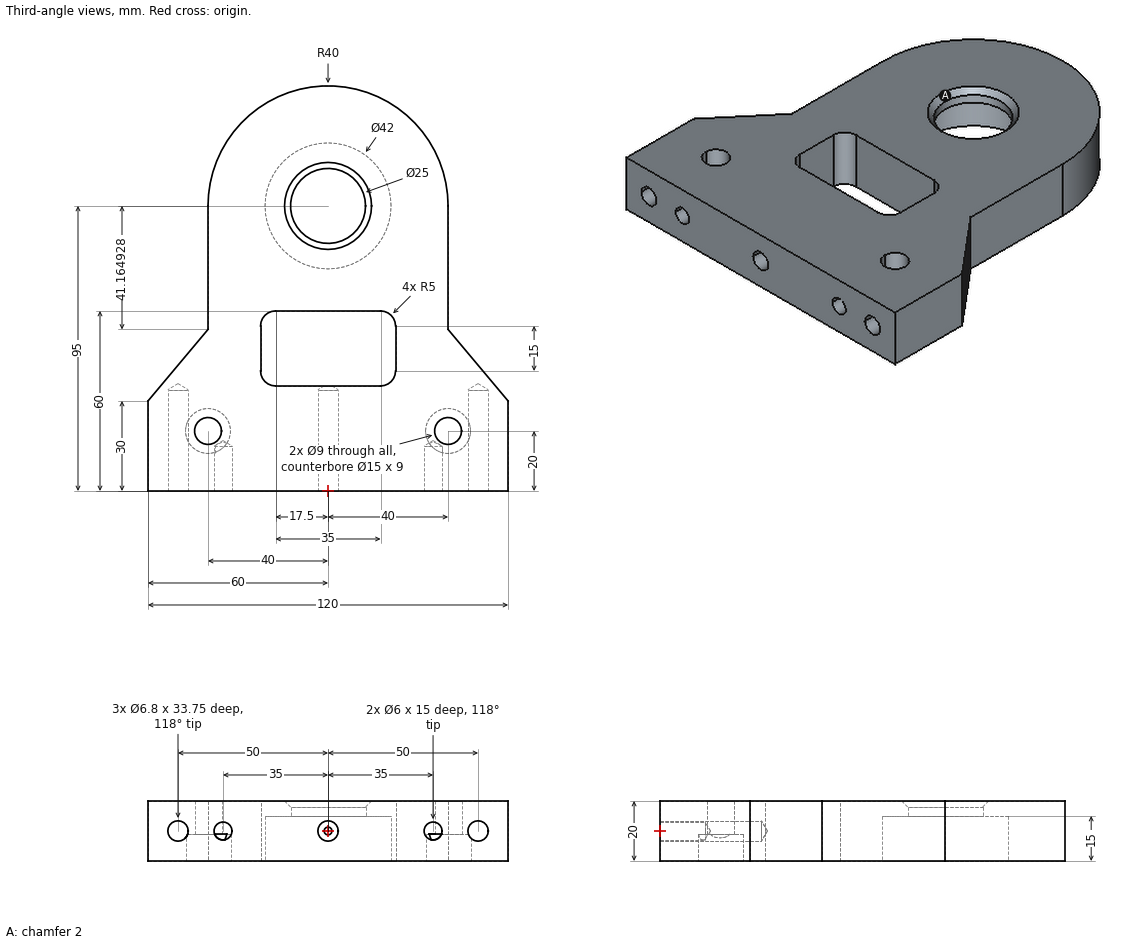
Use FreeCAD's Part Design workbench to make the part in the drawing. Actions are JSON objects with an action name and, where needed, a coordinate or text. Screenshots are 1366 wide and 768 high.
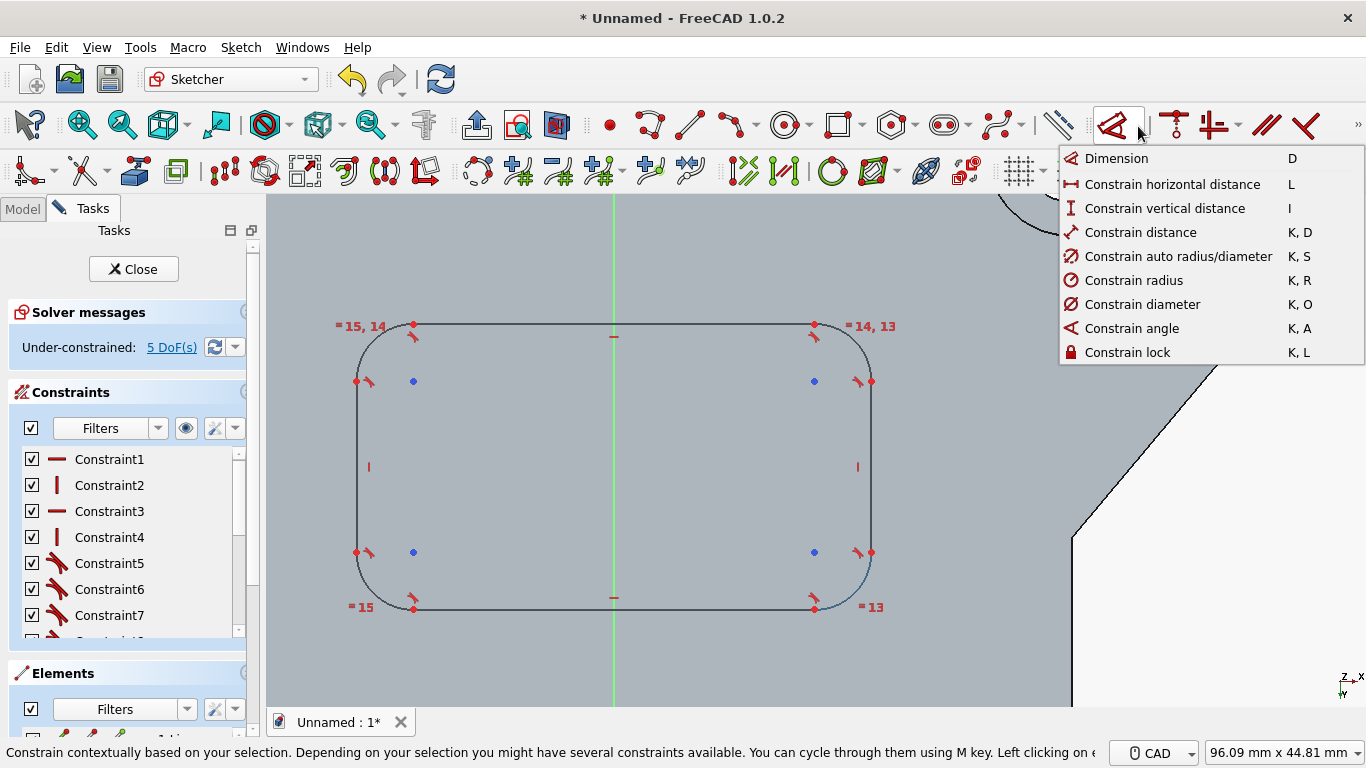
{"action": "left_click", "coordinate": [1212, 280]}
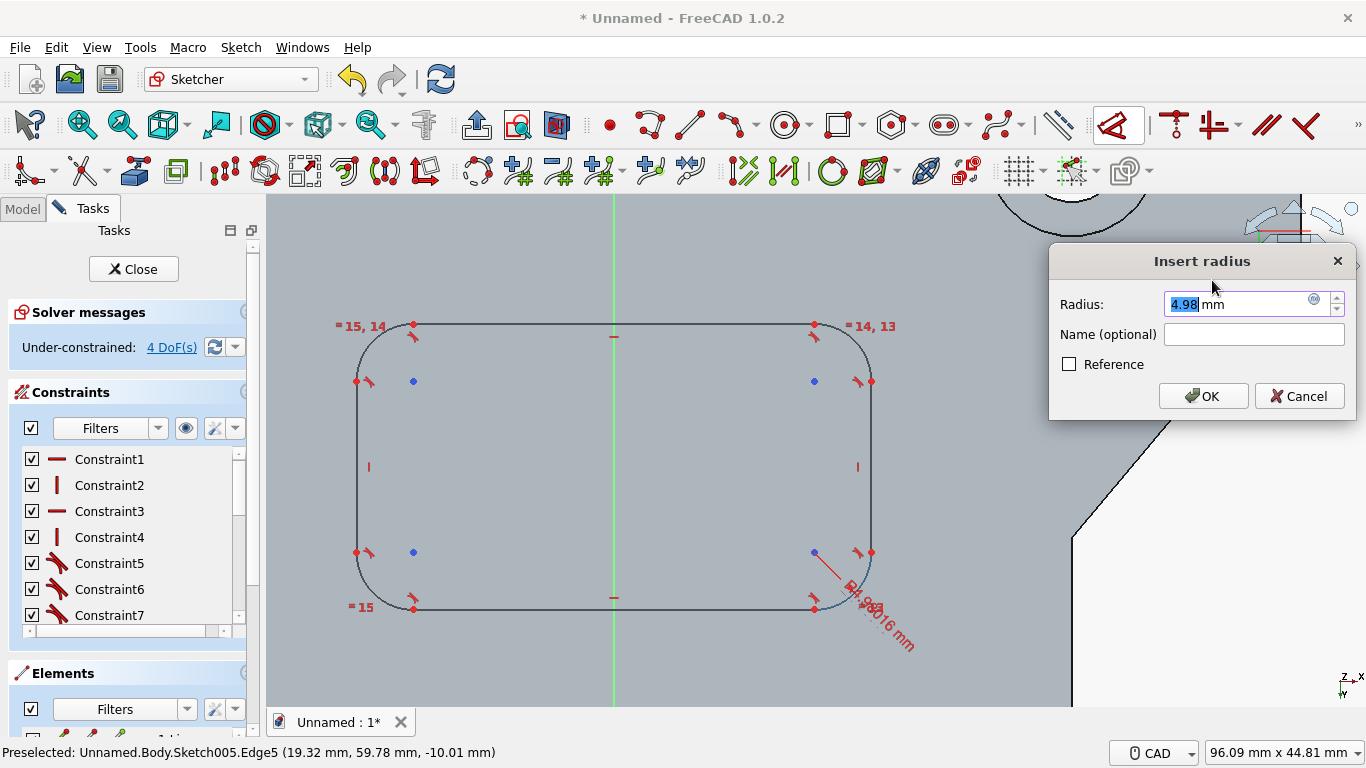
{"action": "type", "text": "5"}
{"action": "key", "text": "Return"}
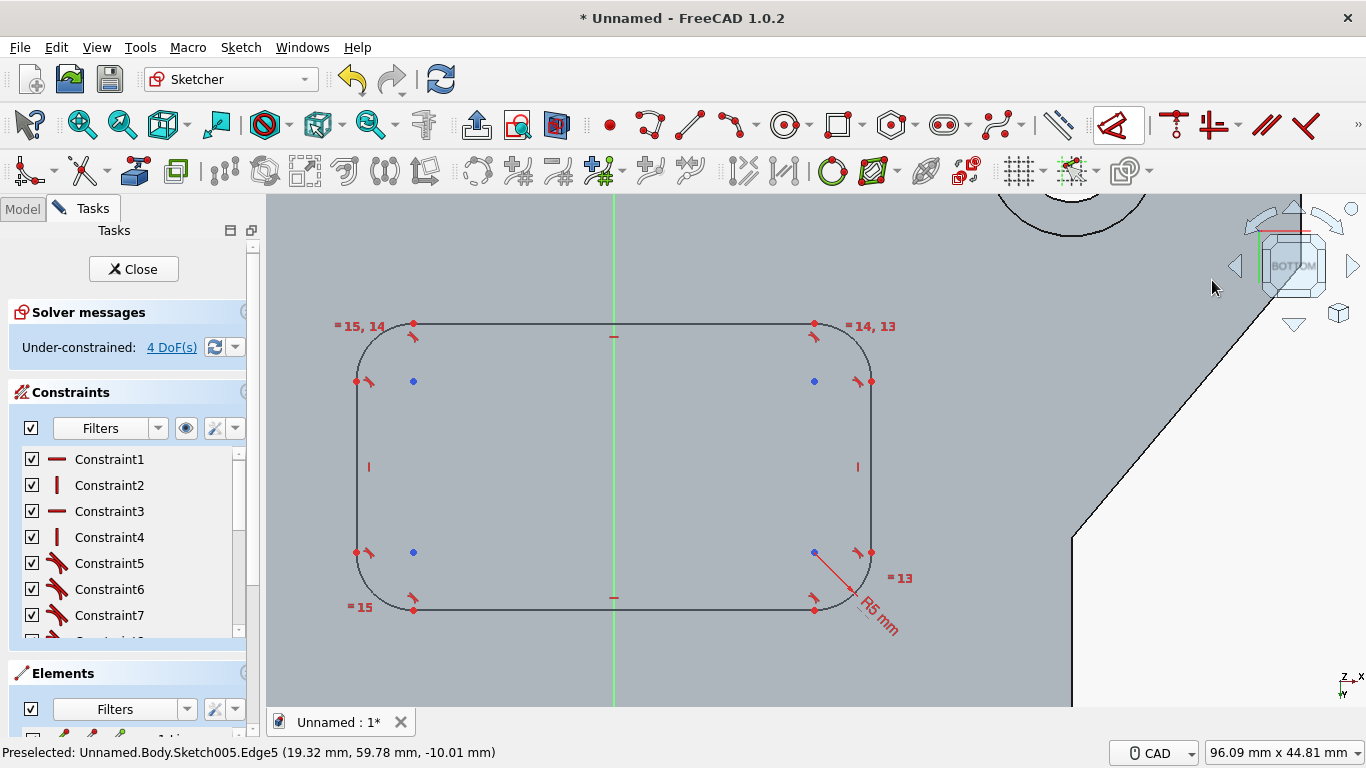
{"action": "left_click", "coordinate": [534, 610]}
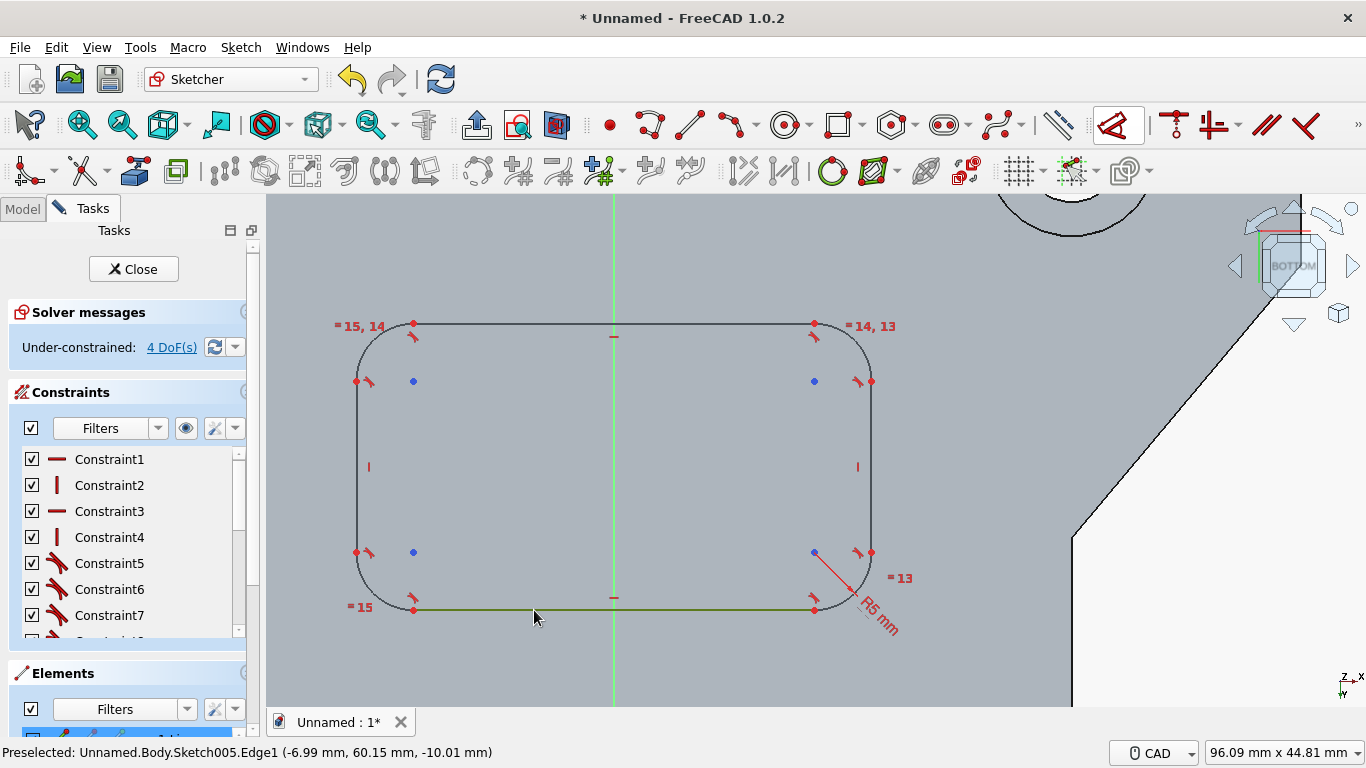
{"action": "key", "text": "l"}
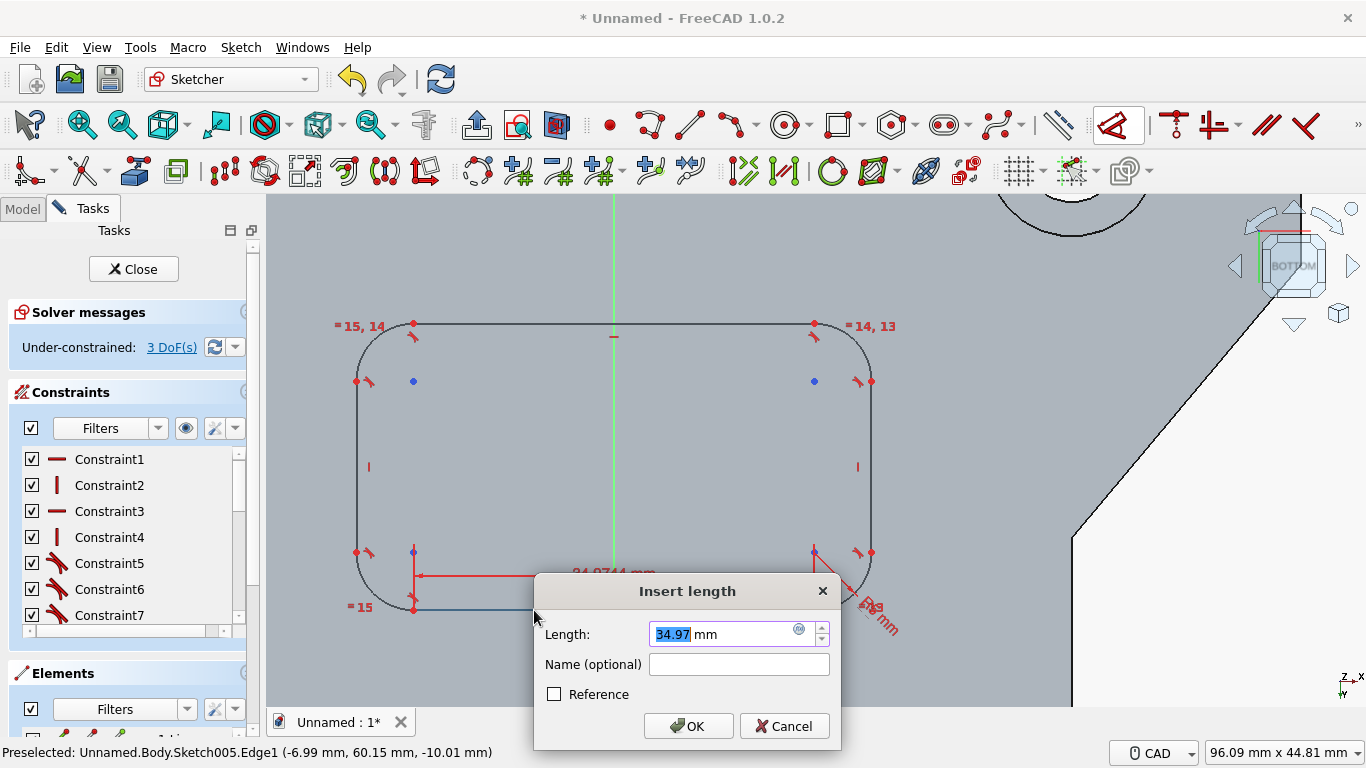
{"action": "type", "text": "35"}
{"action": "key", "text": "Return"}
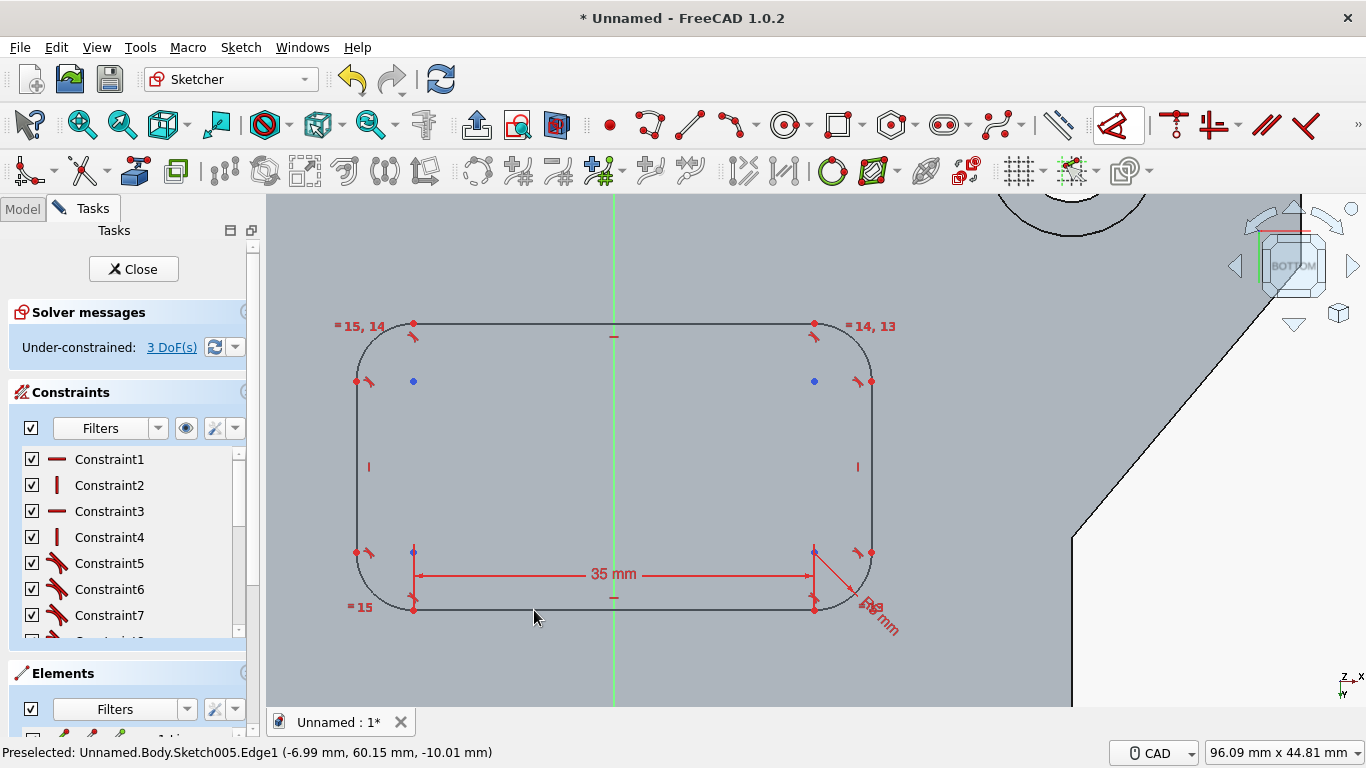
{"action": "left_click", "coordinate": [872, 501]}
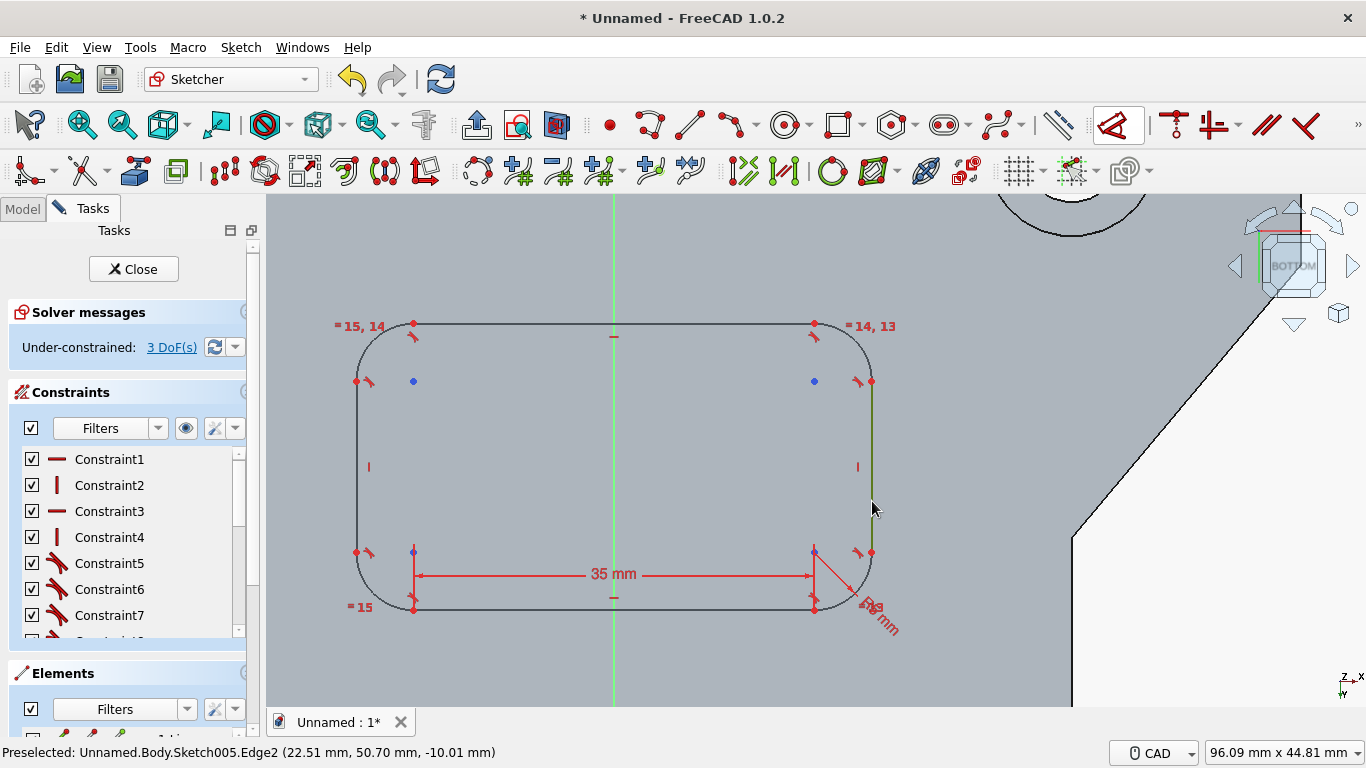
{"action": "left_click", "coordinate": [1138, 126]}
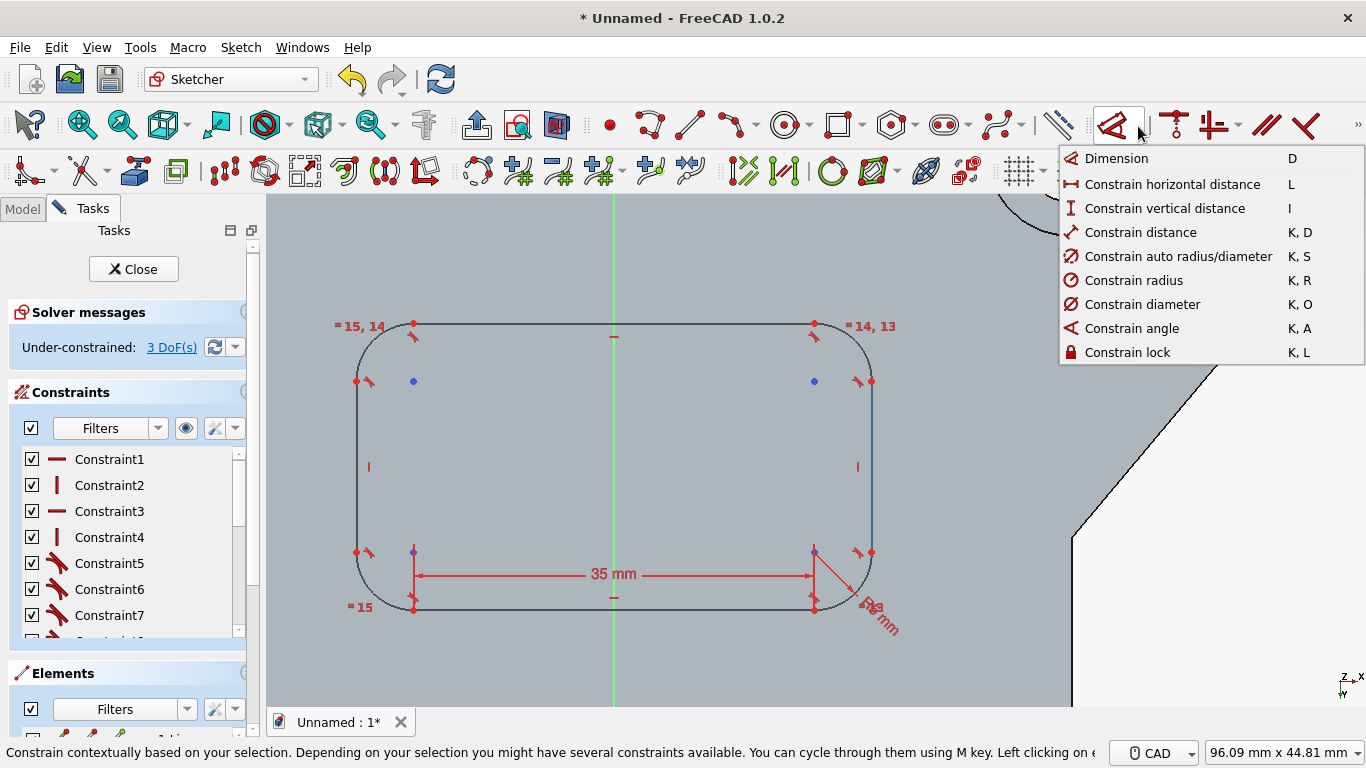
{"action": "left_click", "coordinate": [1212, 208]}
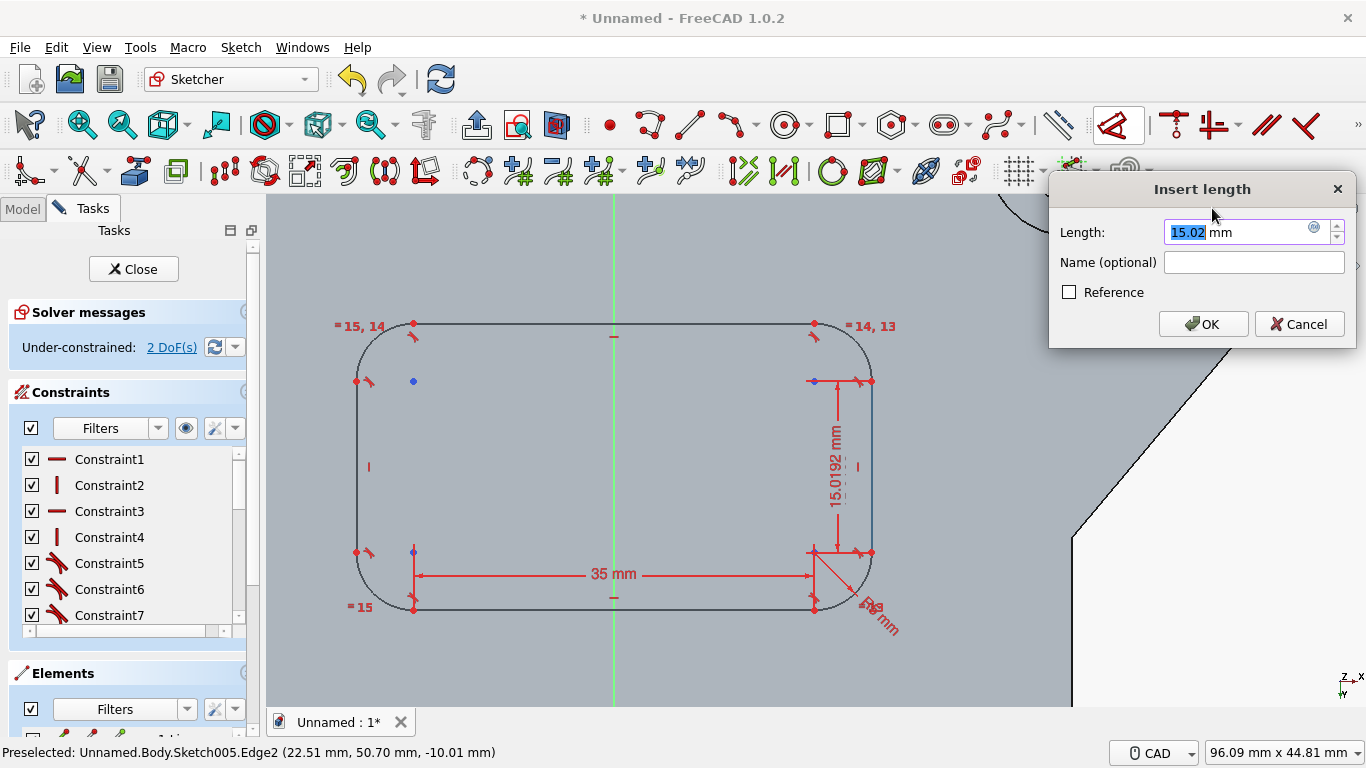
{"action": "type", "text": "15"}
{"action": "key", "text": "Return"}